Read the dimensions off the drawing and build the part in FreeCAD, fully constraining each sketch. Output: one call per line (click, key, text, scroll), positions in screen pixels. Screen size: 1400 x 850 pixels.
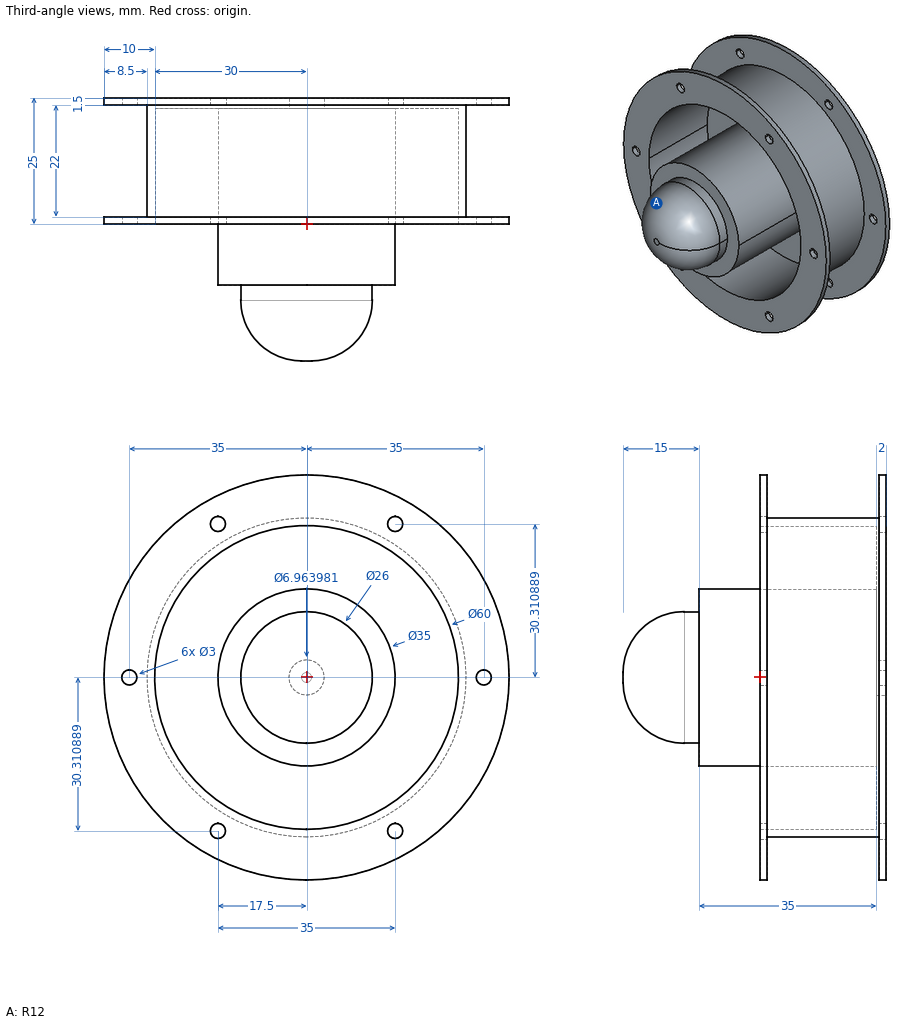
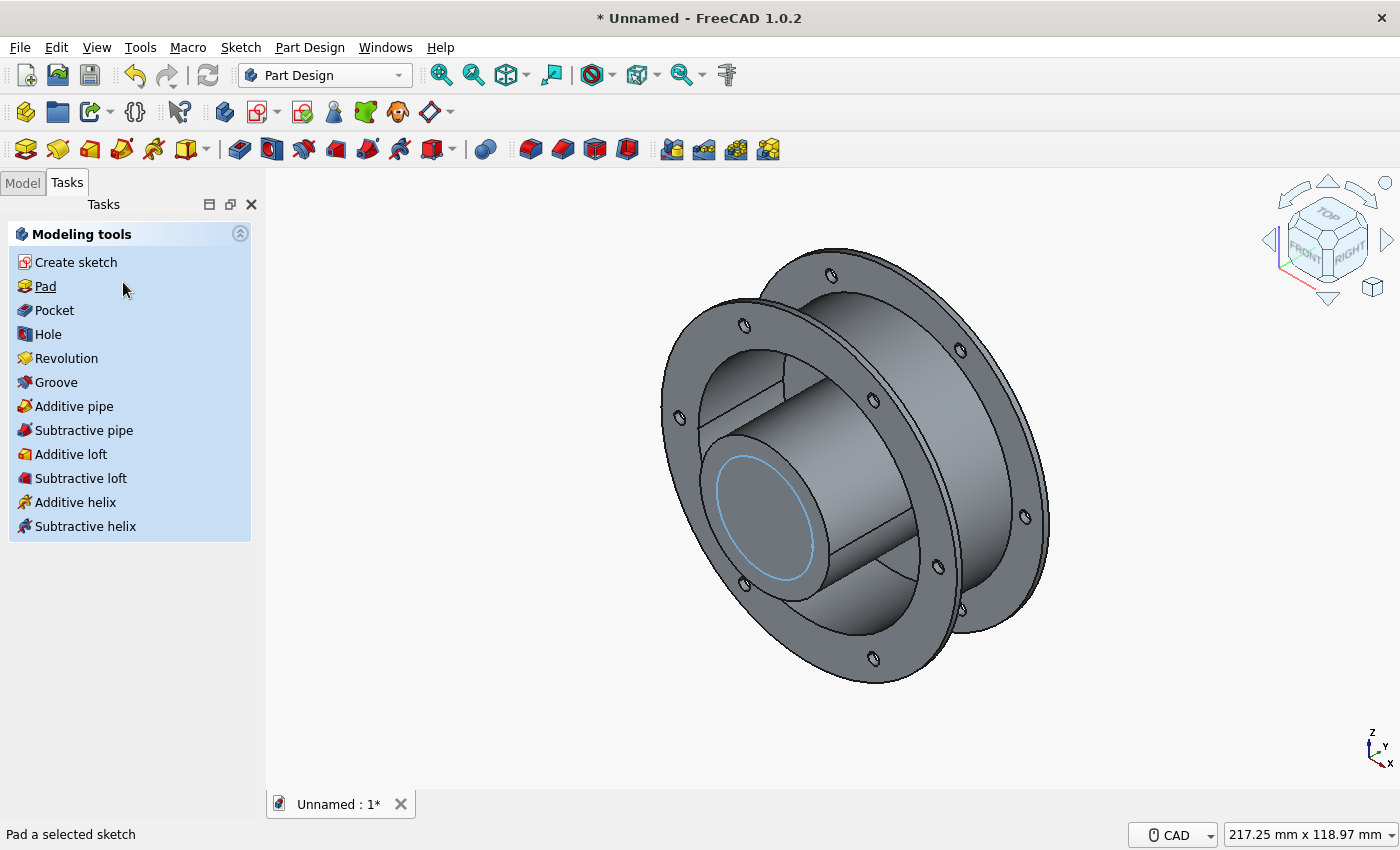
click(26, 150)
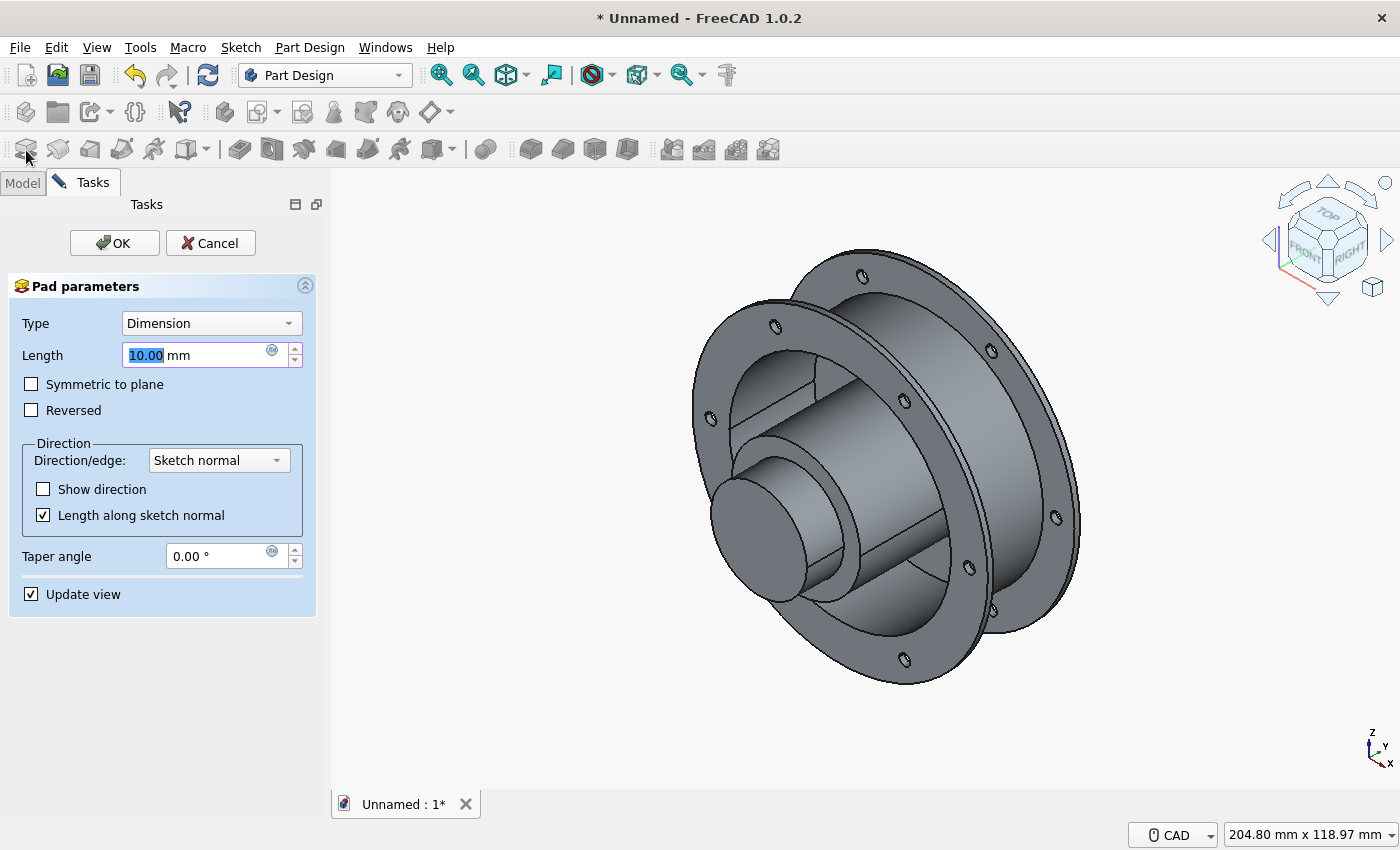
text(15)
key(Tab)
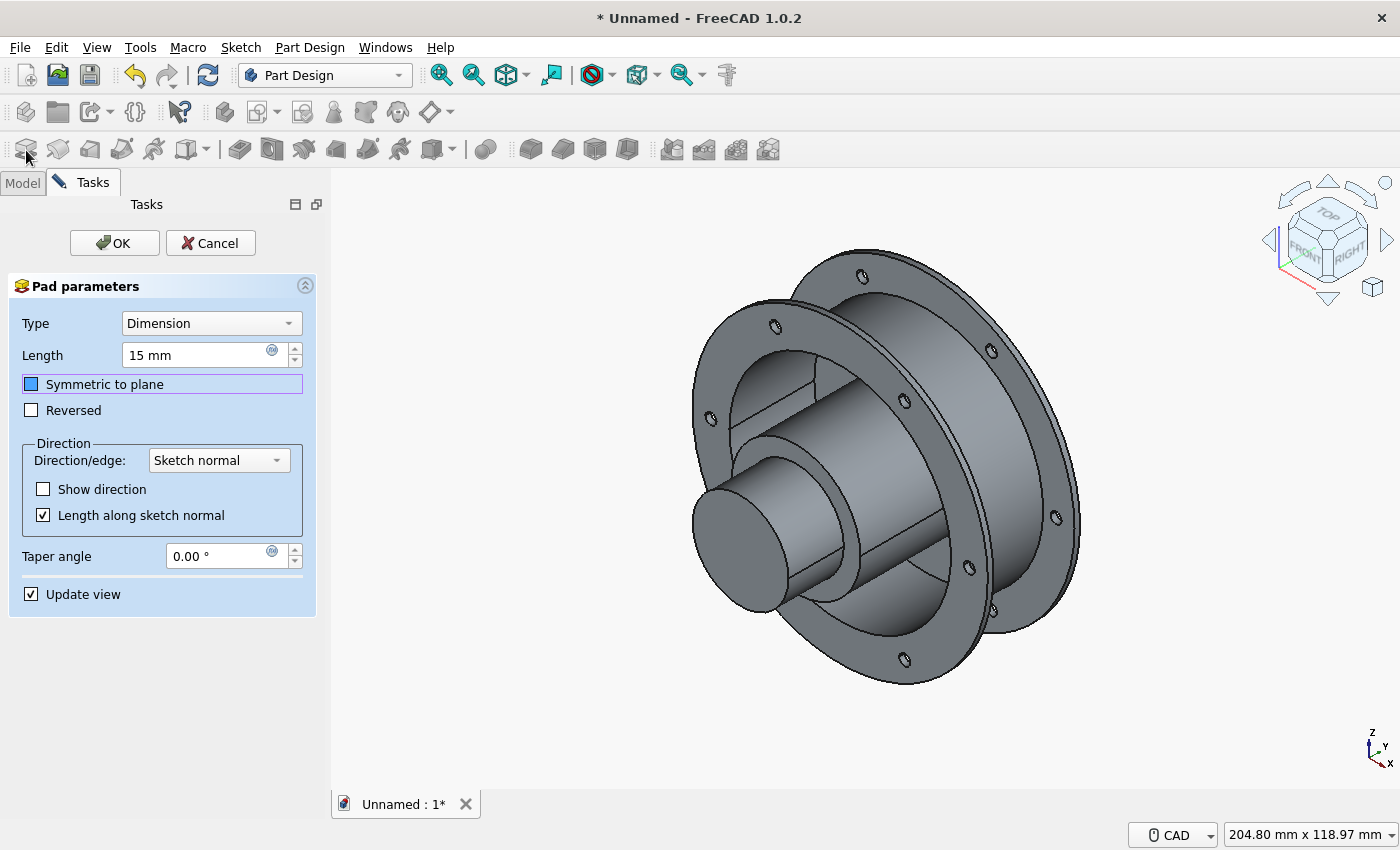
click(115, 243)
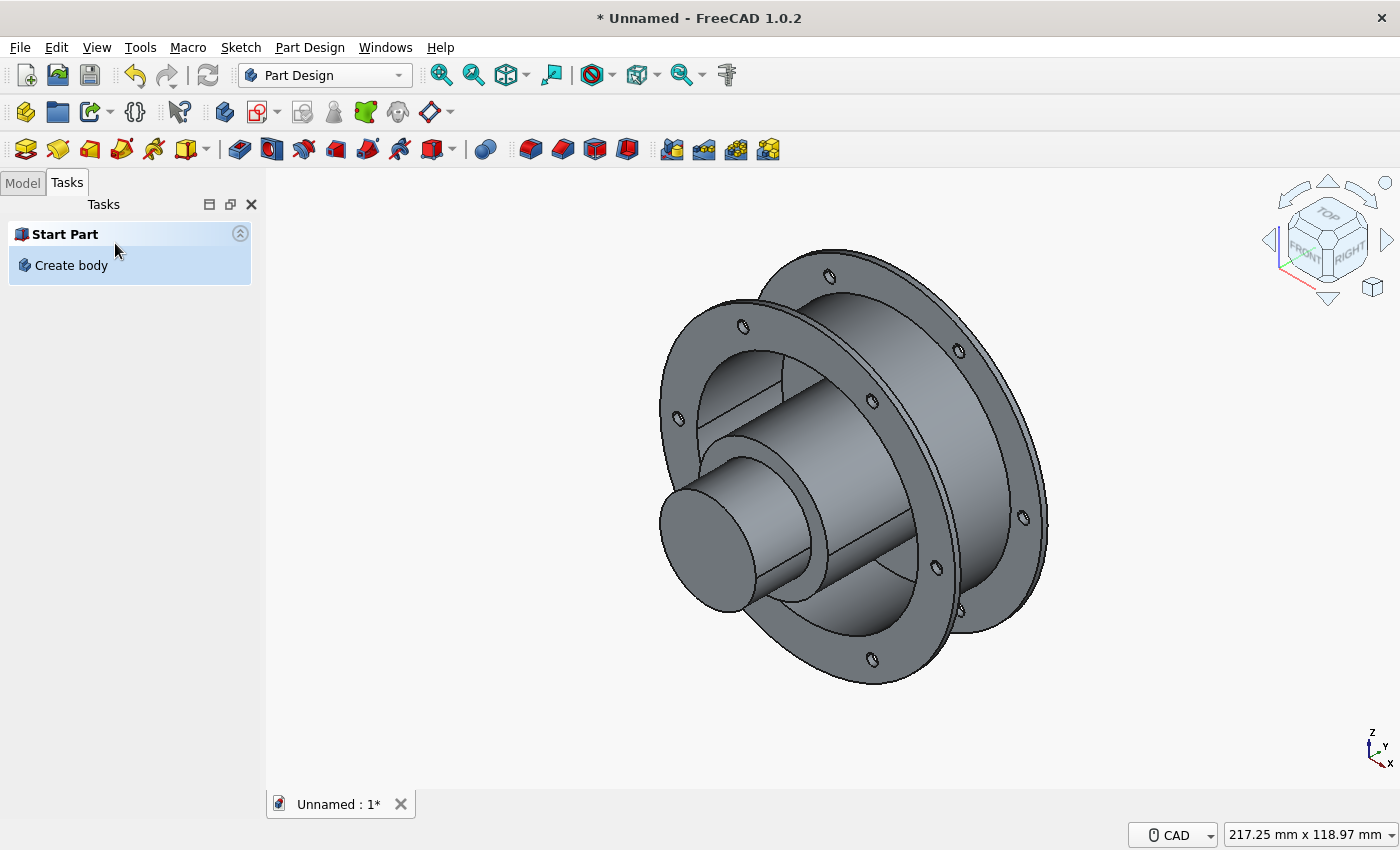
click(442, 76)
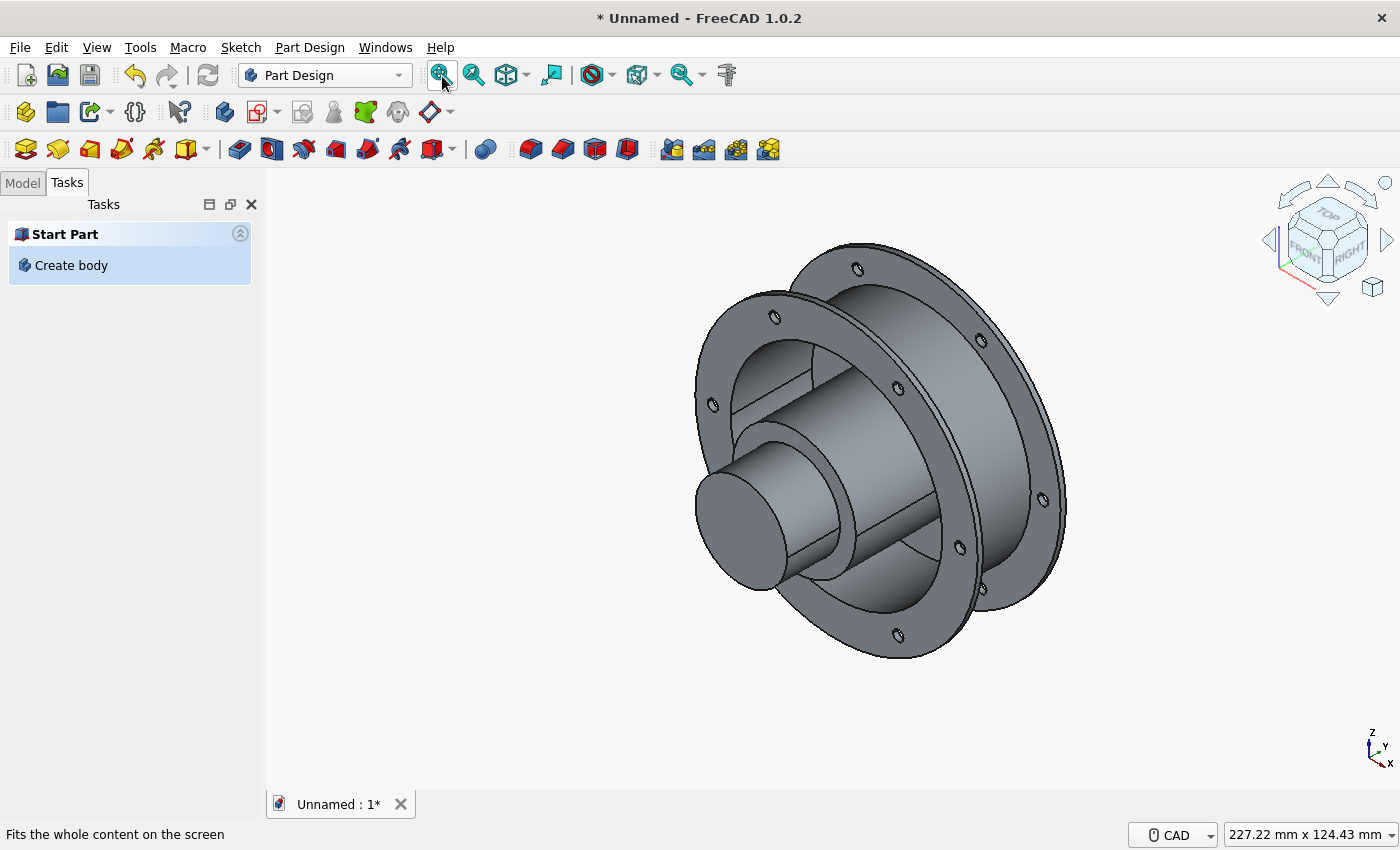
click(727, 472)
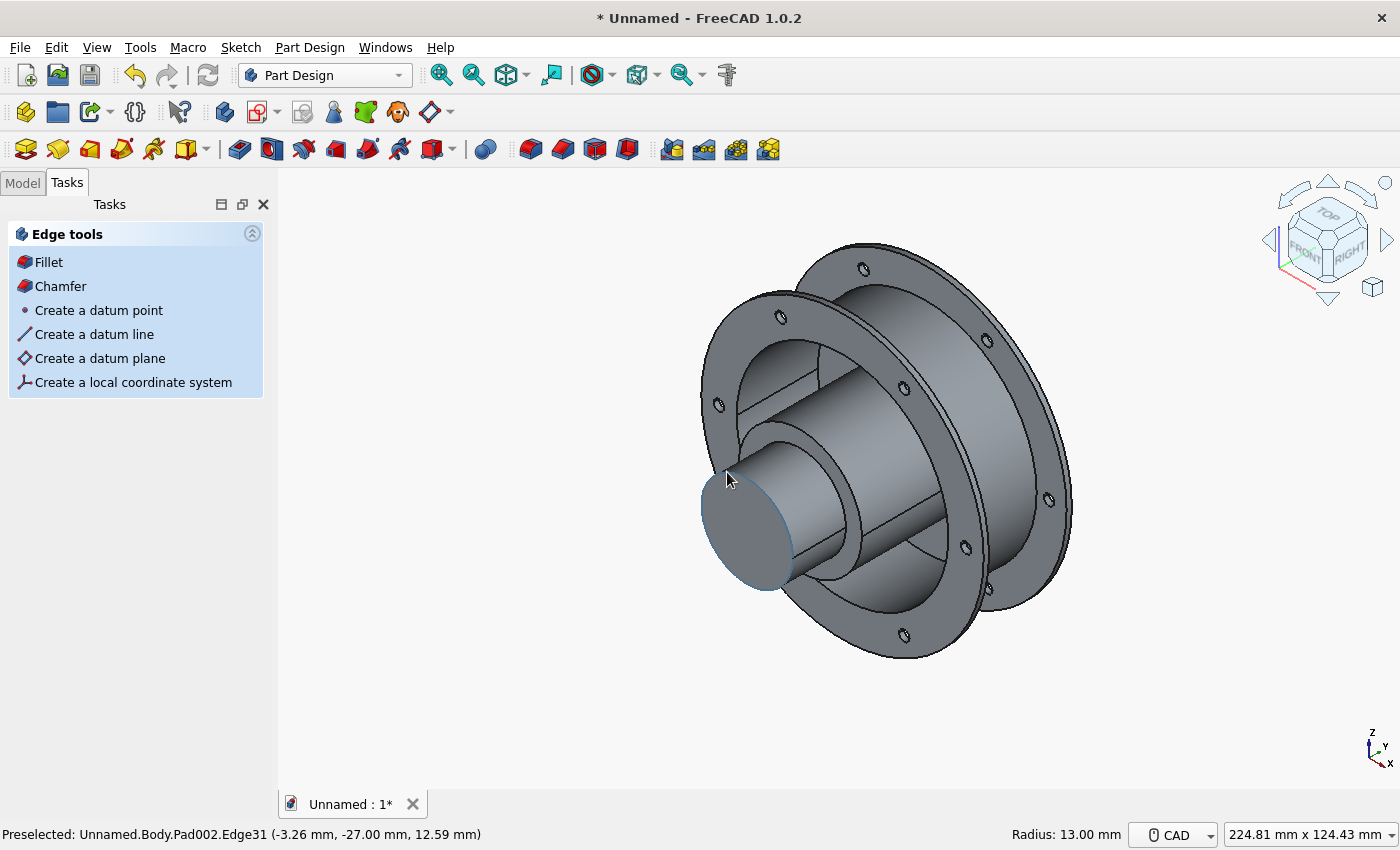
click(532, 150)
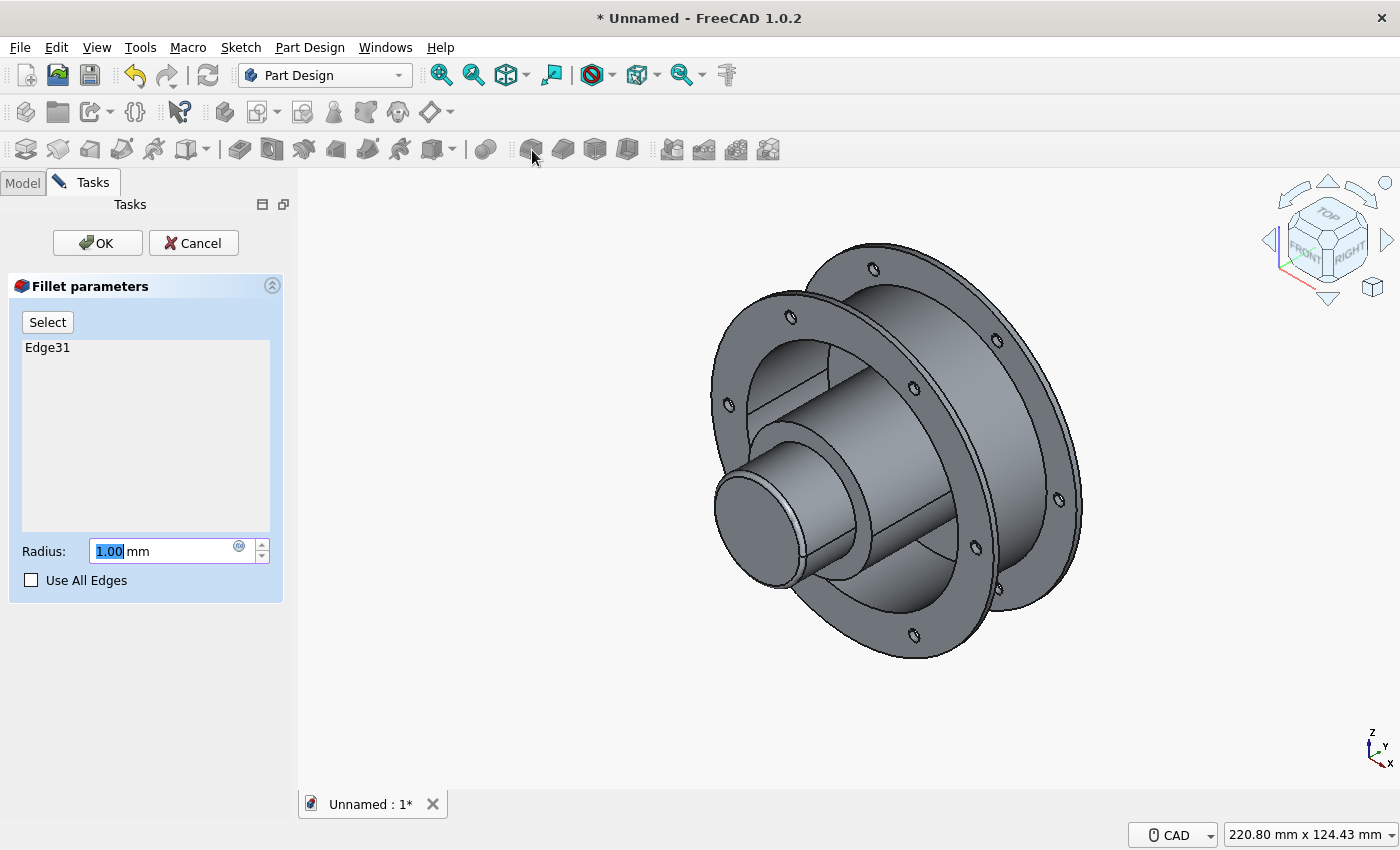
text(12)
key(Tab)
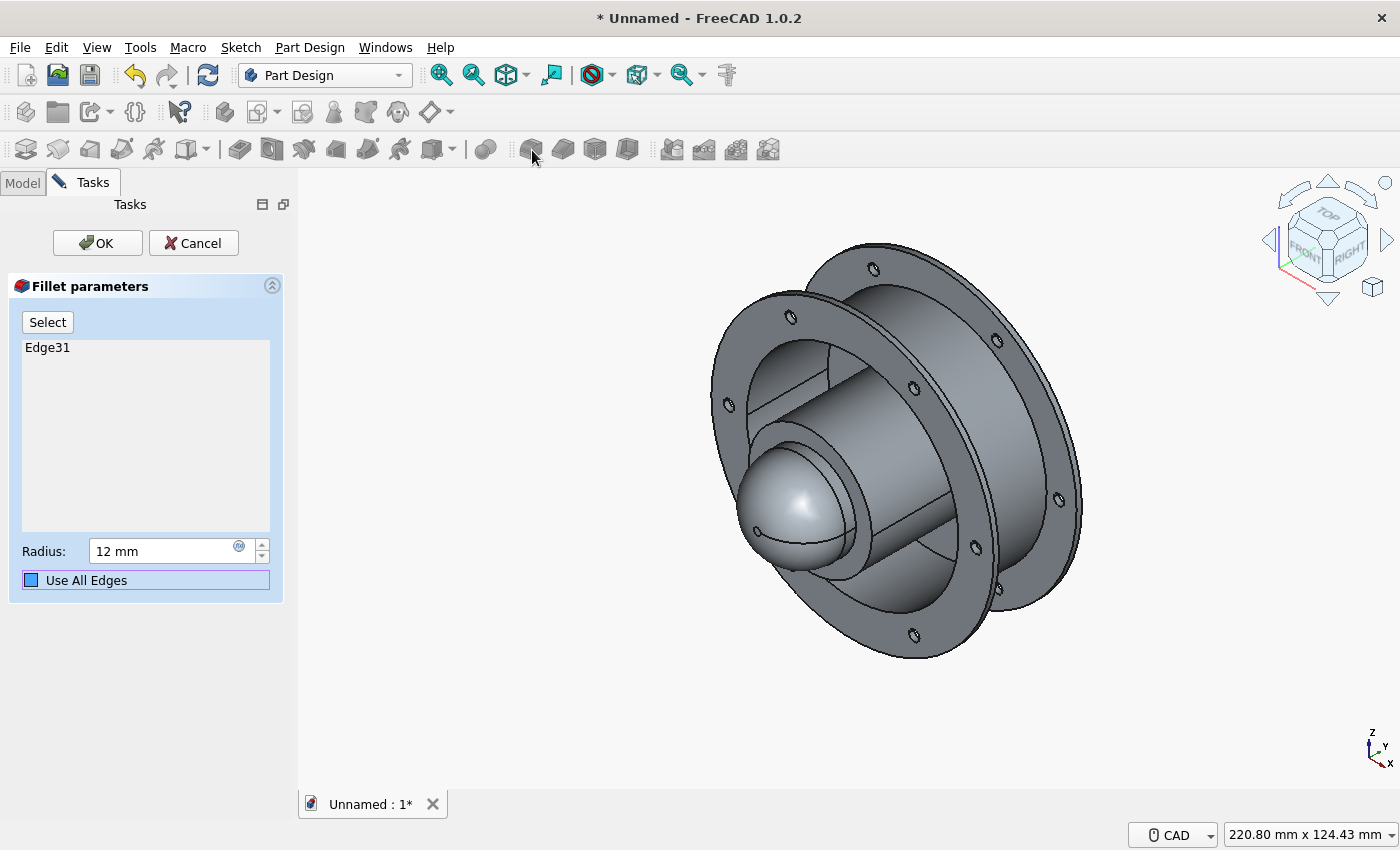
click(98, 243)